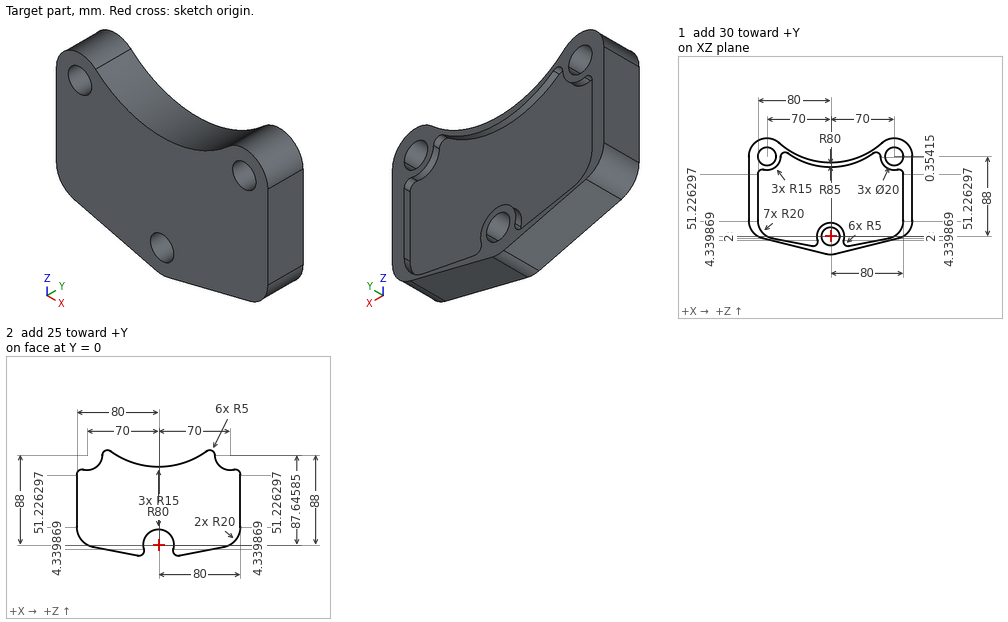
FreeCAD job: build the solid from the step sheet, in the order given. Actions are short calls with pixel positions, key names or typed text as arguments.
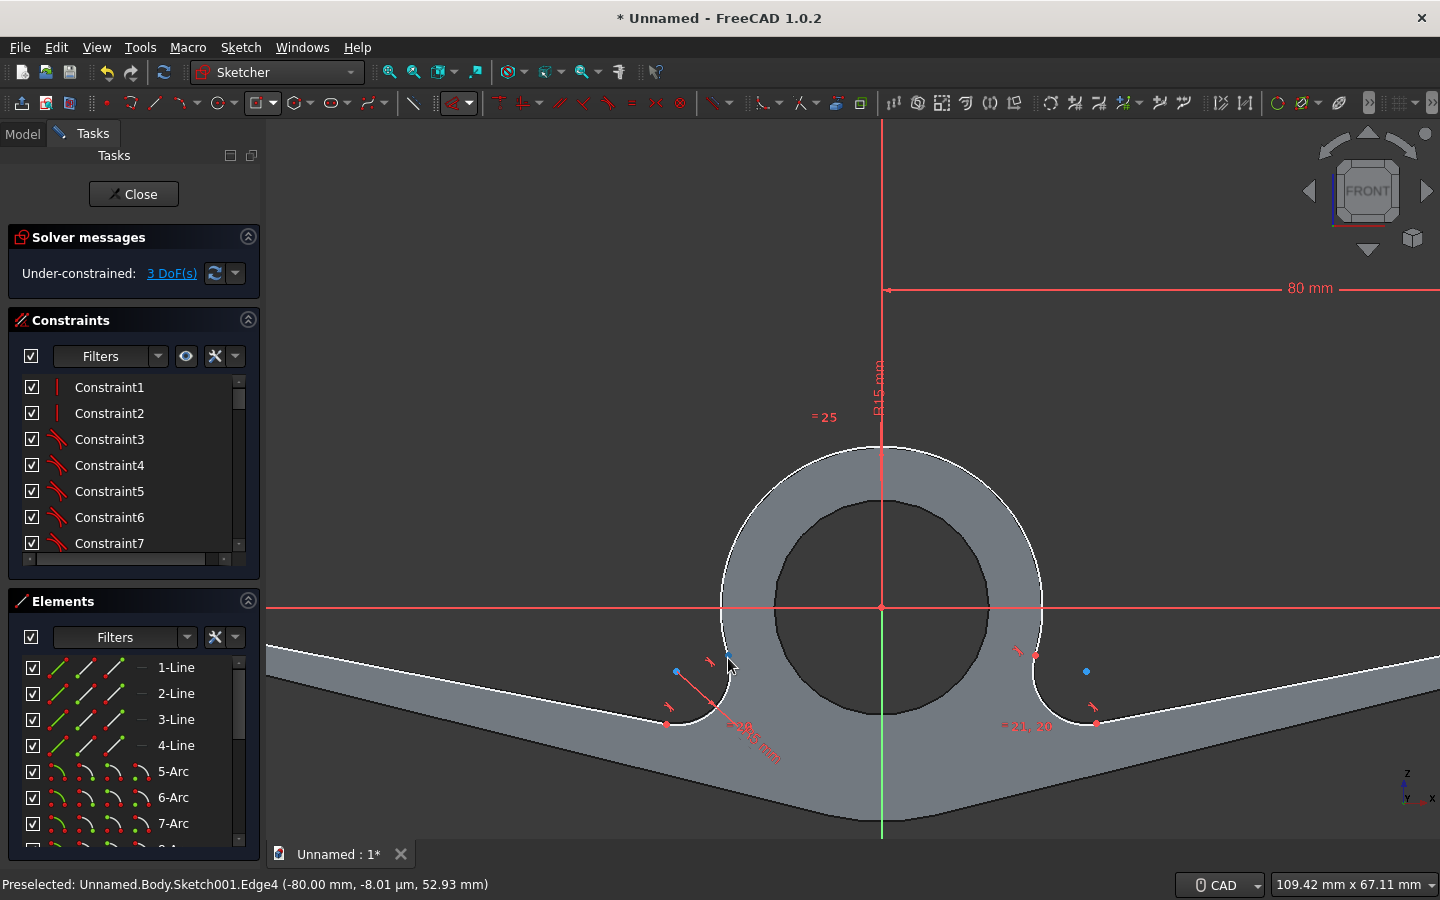
click(728, 656)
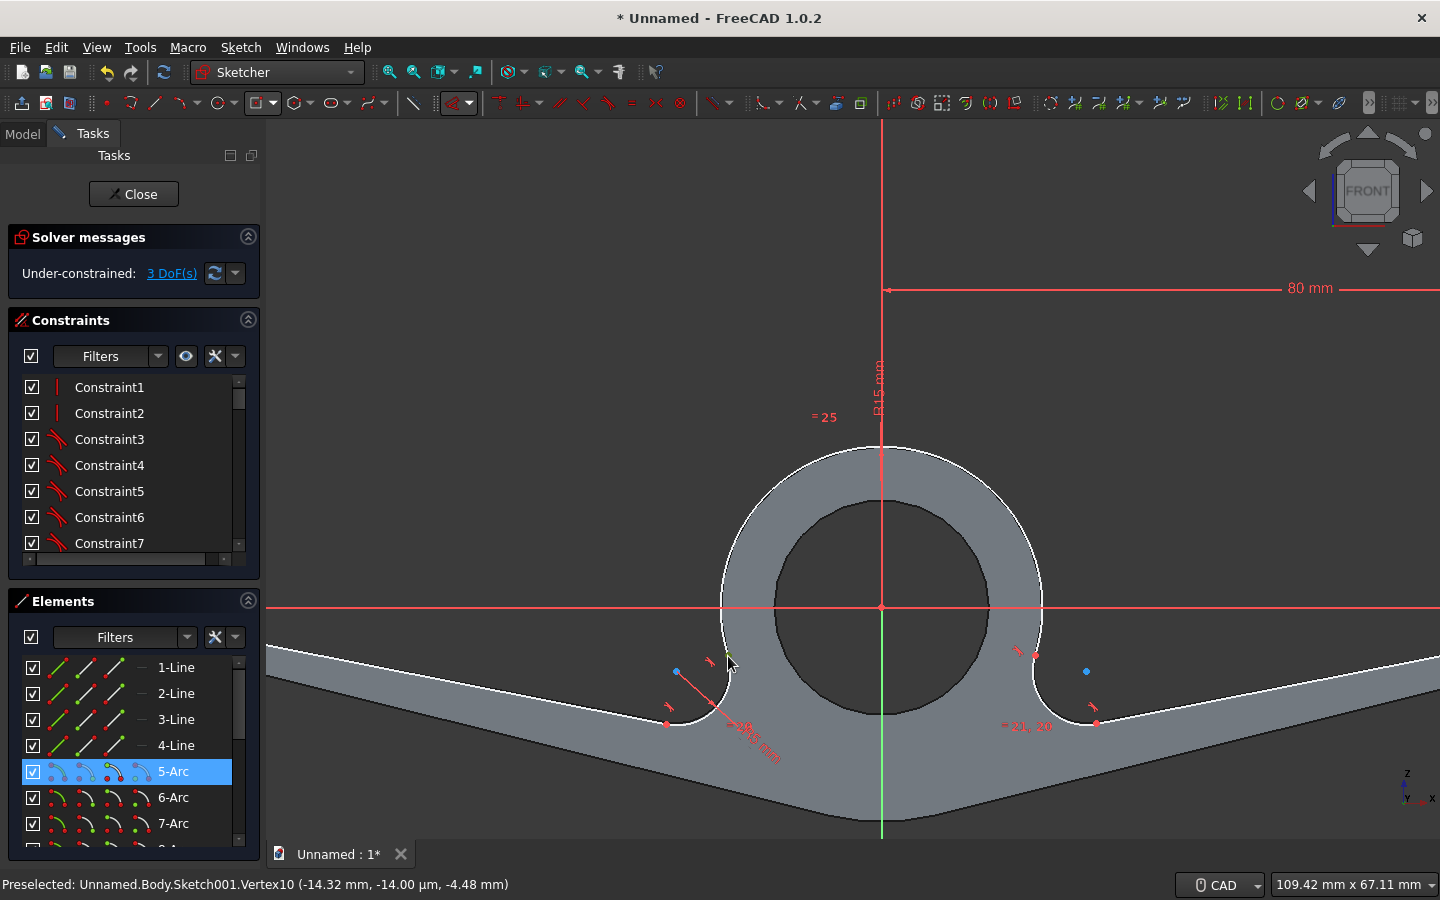
key(i)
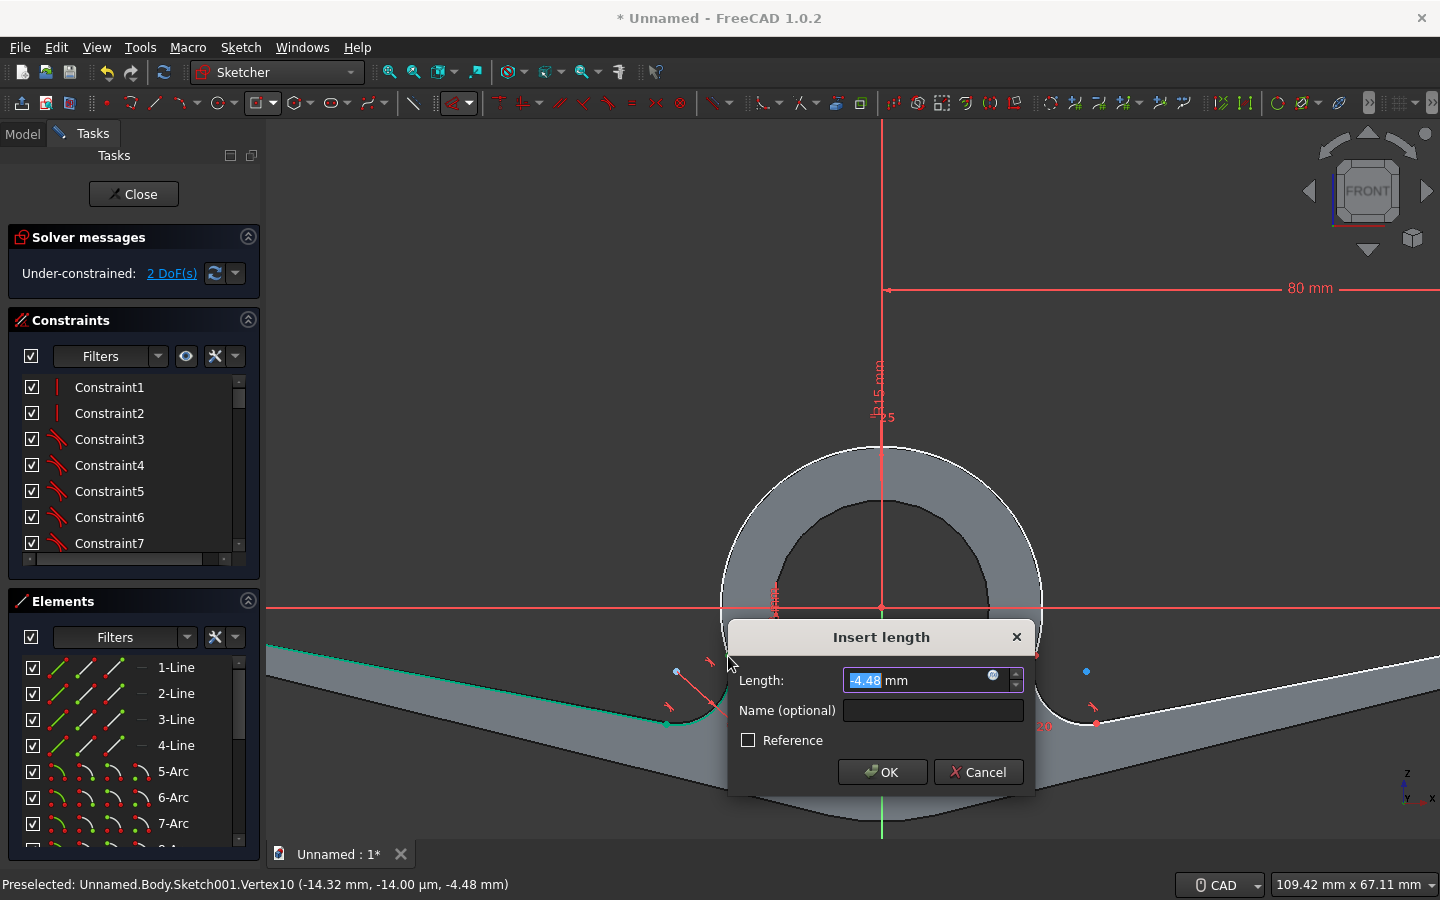
text(-4.339869)
key(Return)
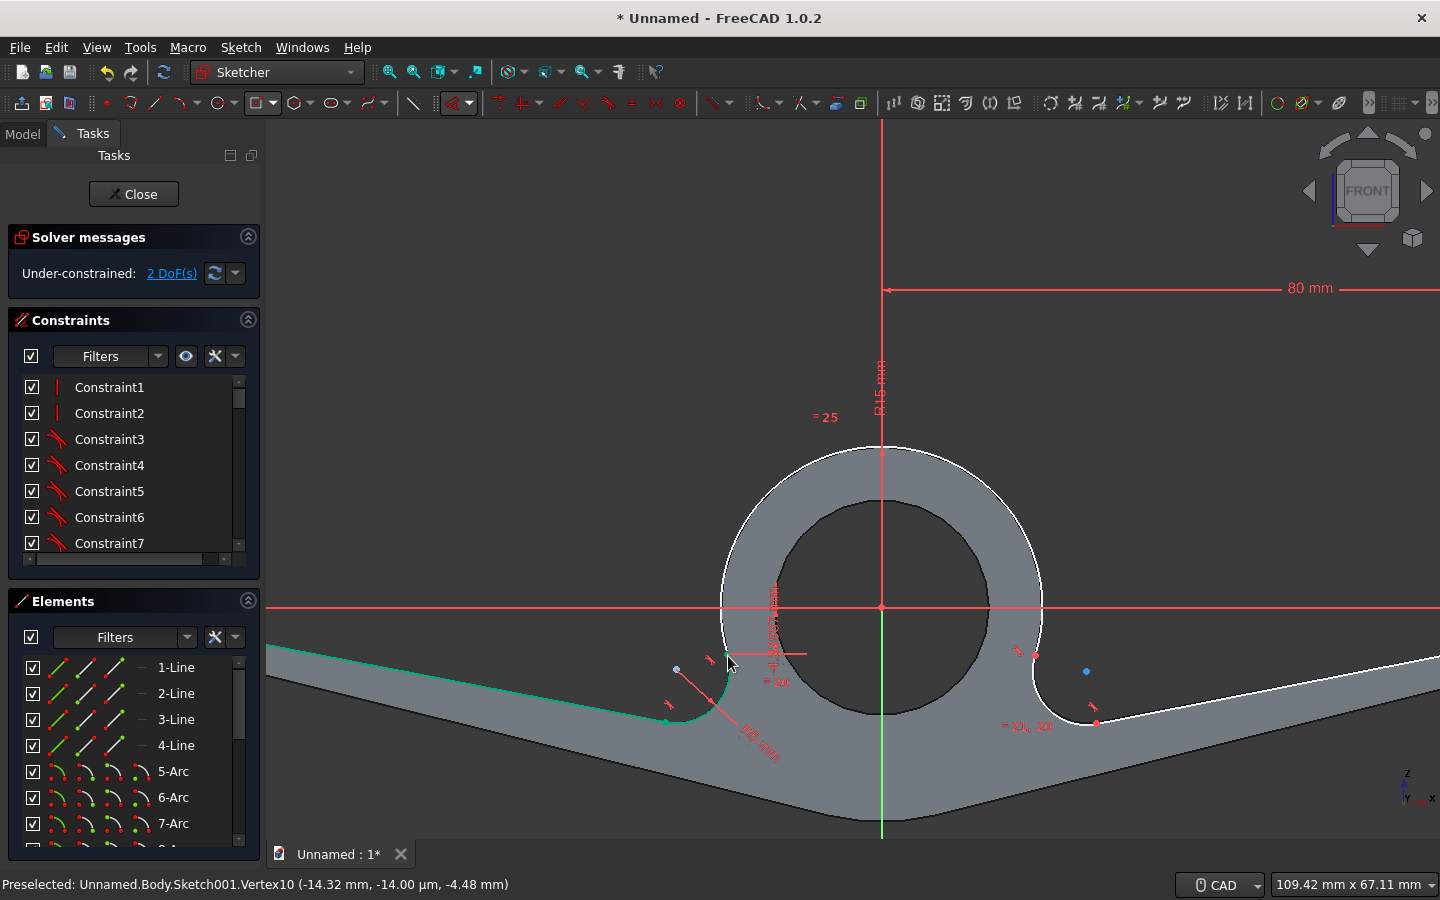
click(1035, 655)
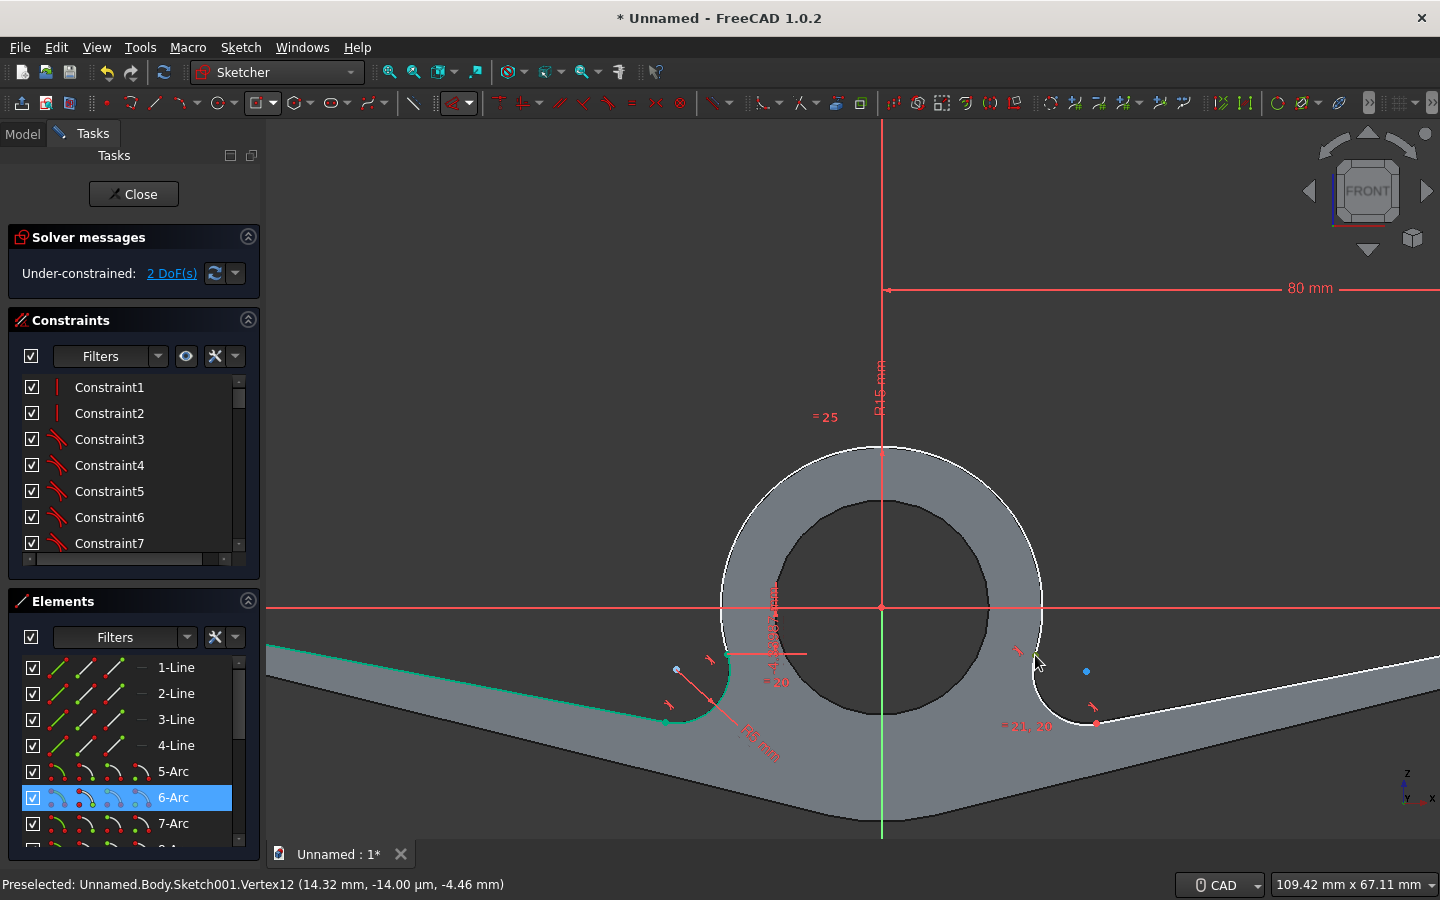
key(i)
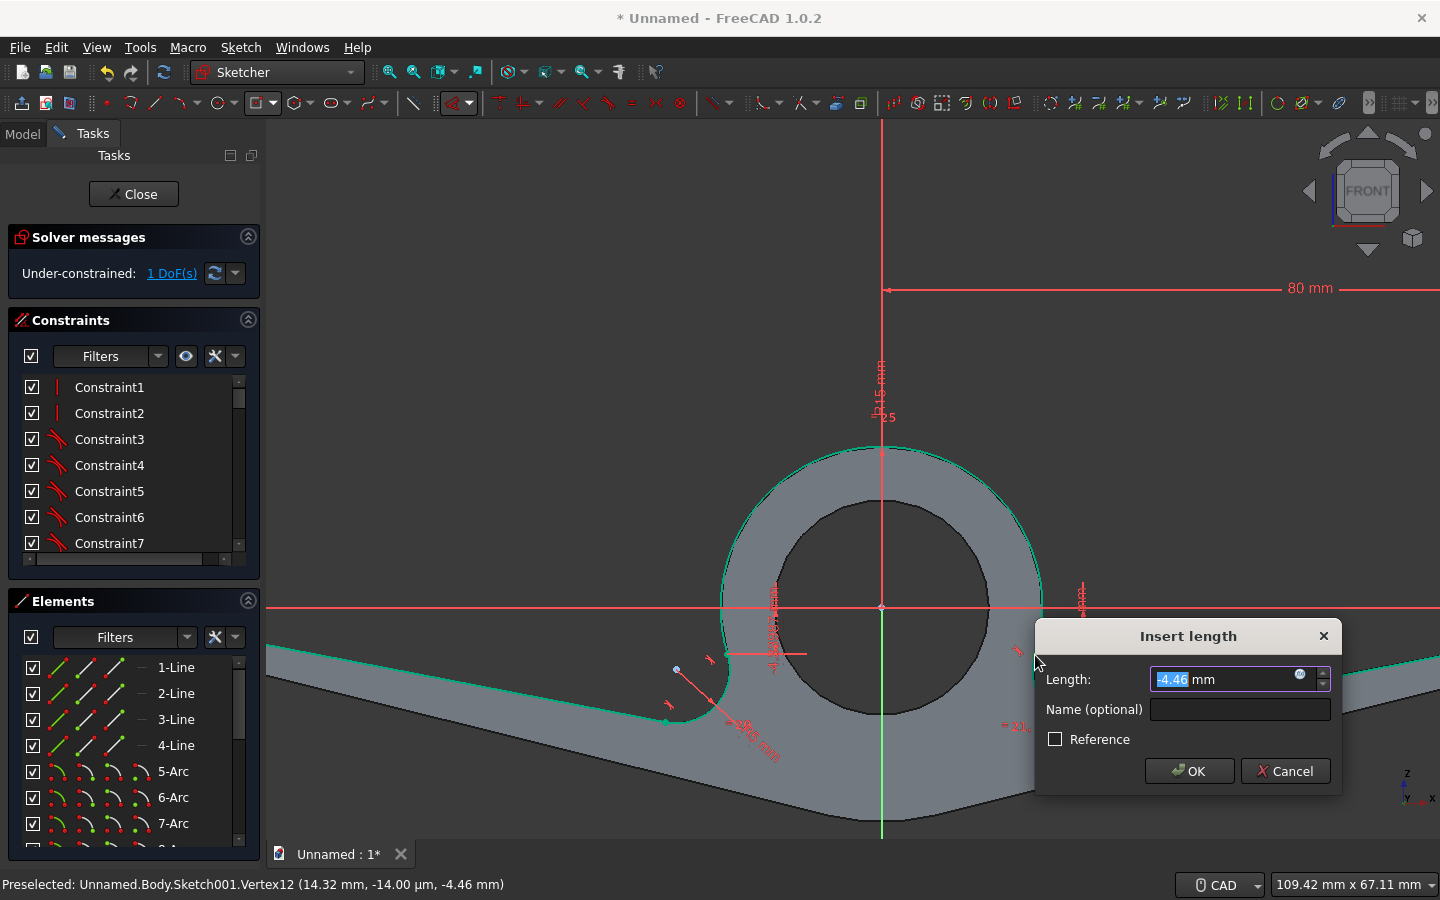
text(-4.339869)
key(Return)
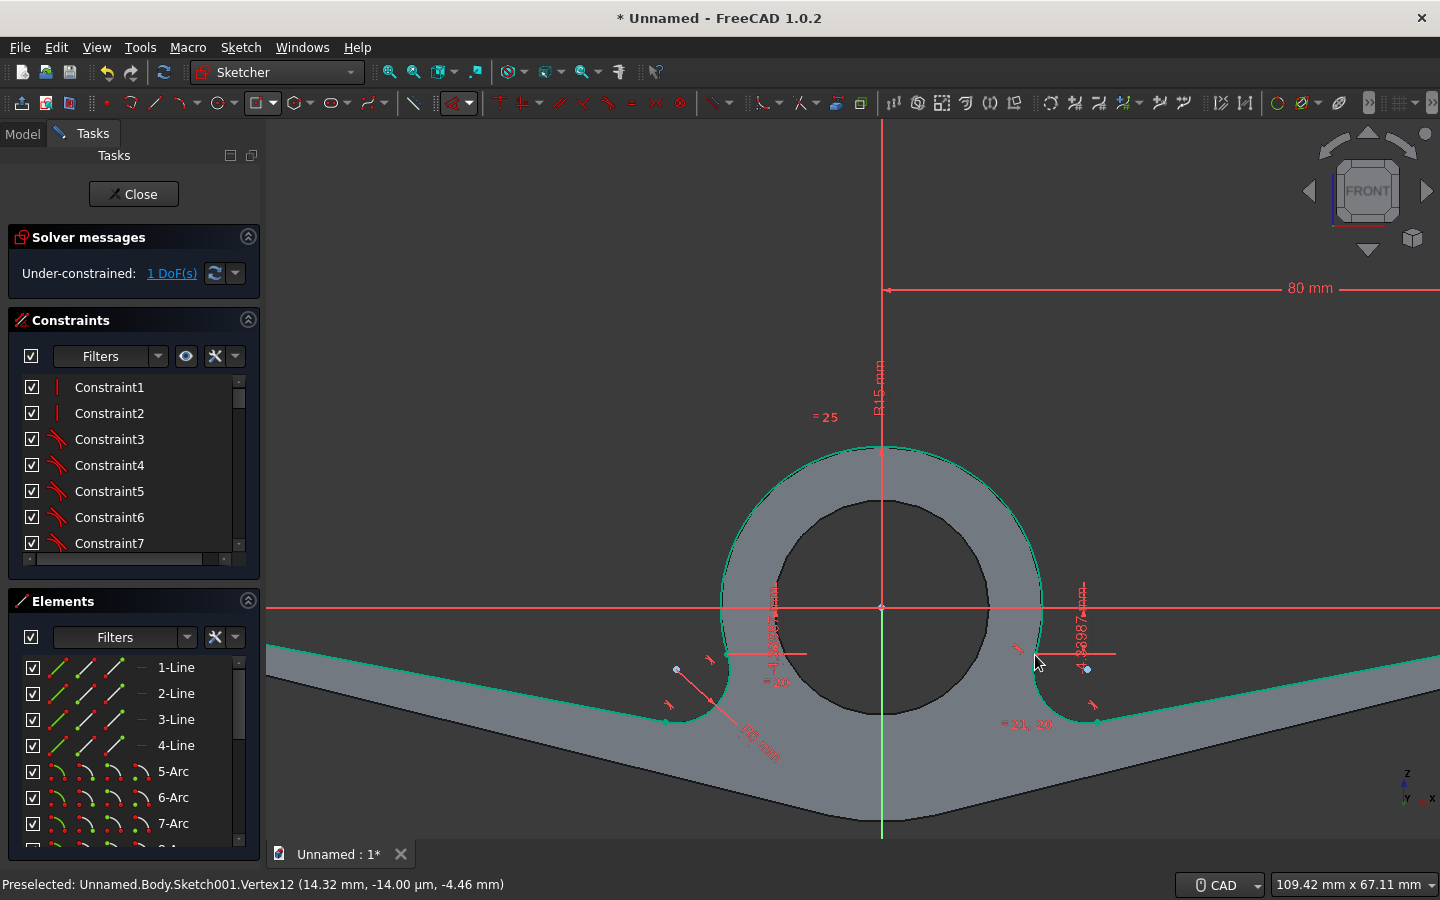
scroll(728, 658, down, 5)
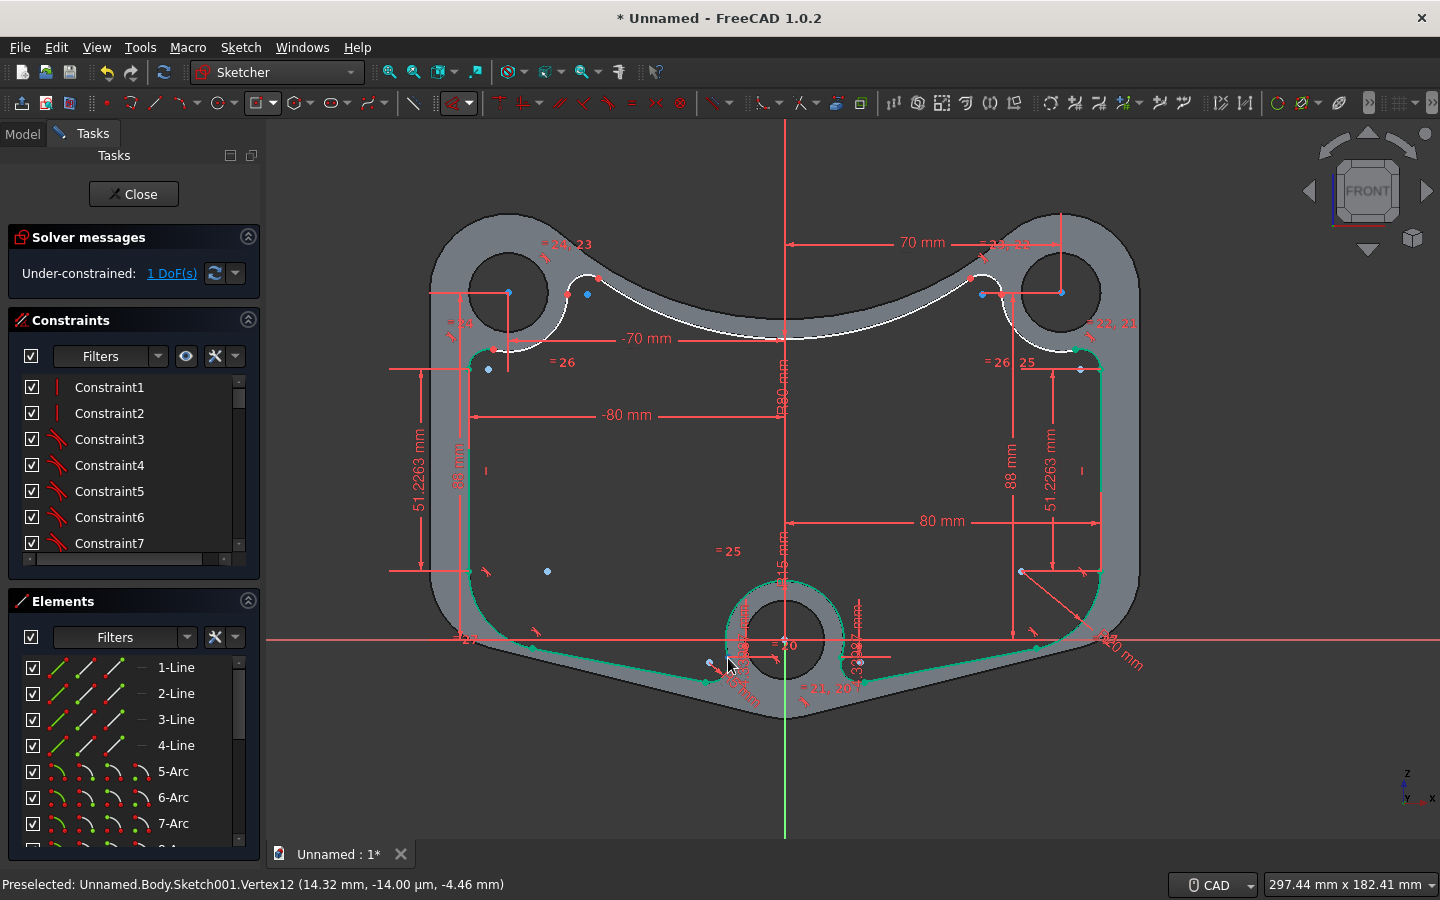
click(1002, 294)